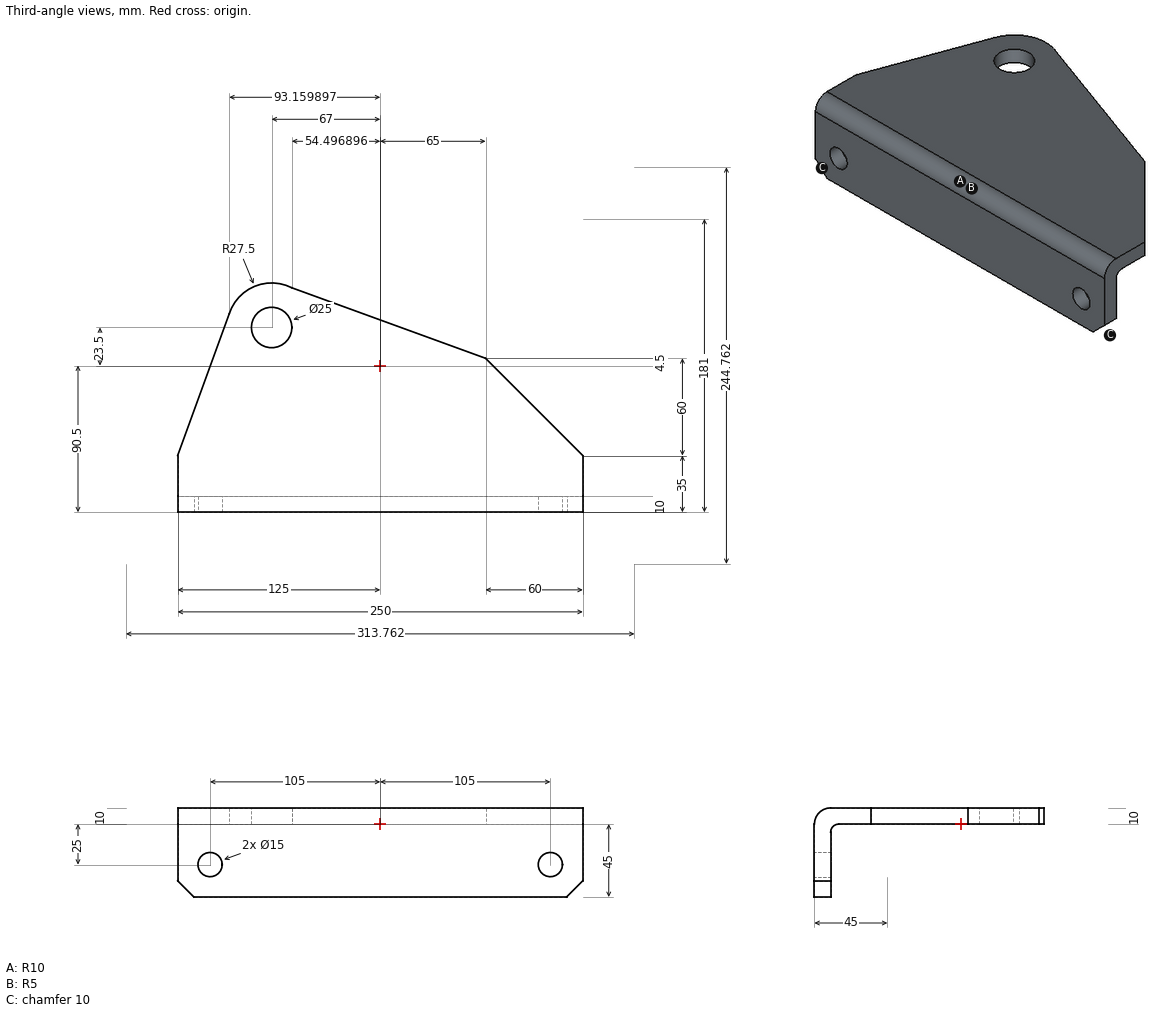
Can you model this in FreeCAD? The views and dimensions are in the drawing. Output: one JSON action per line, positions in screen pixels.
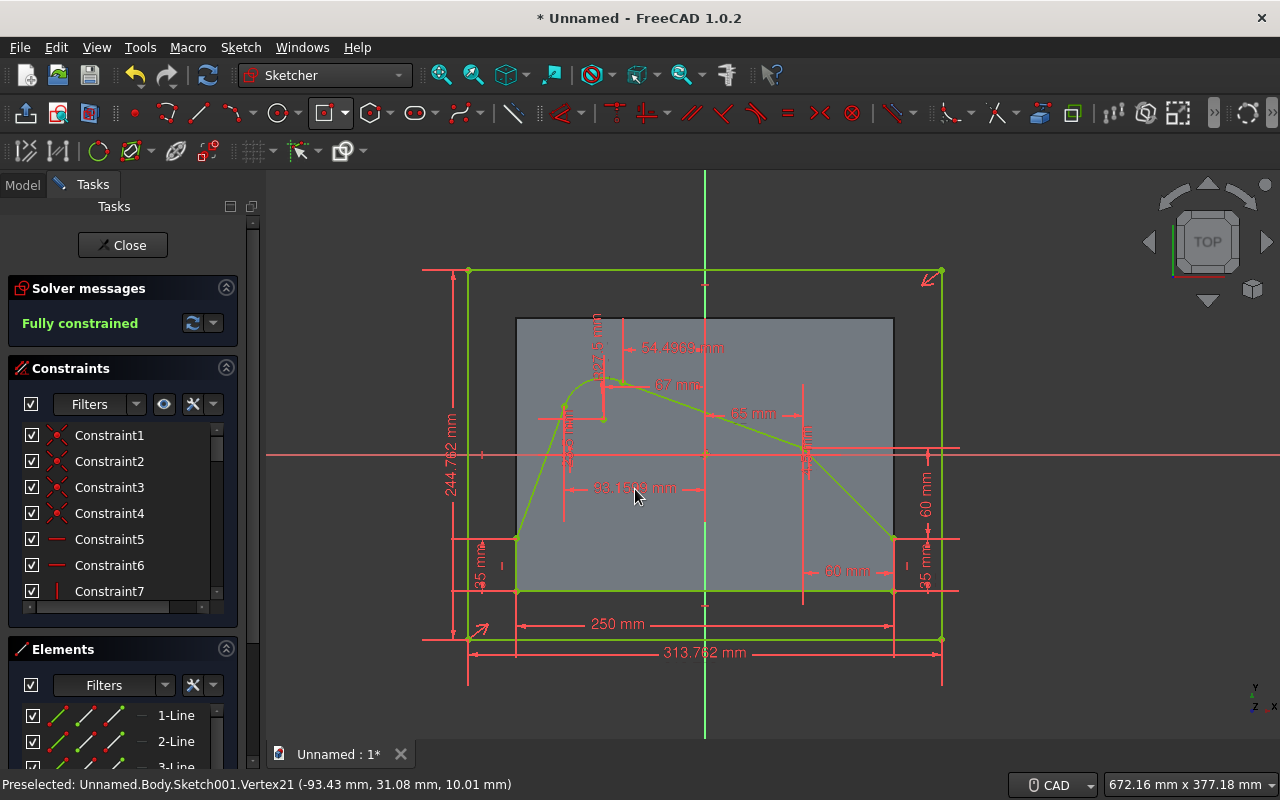
{"action": "left_click", "coordinate": [123, 245]}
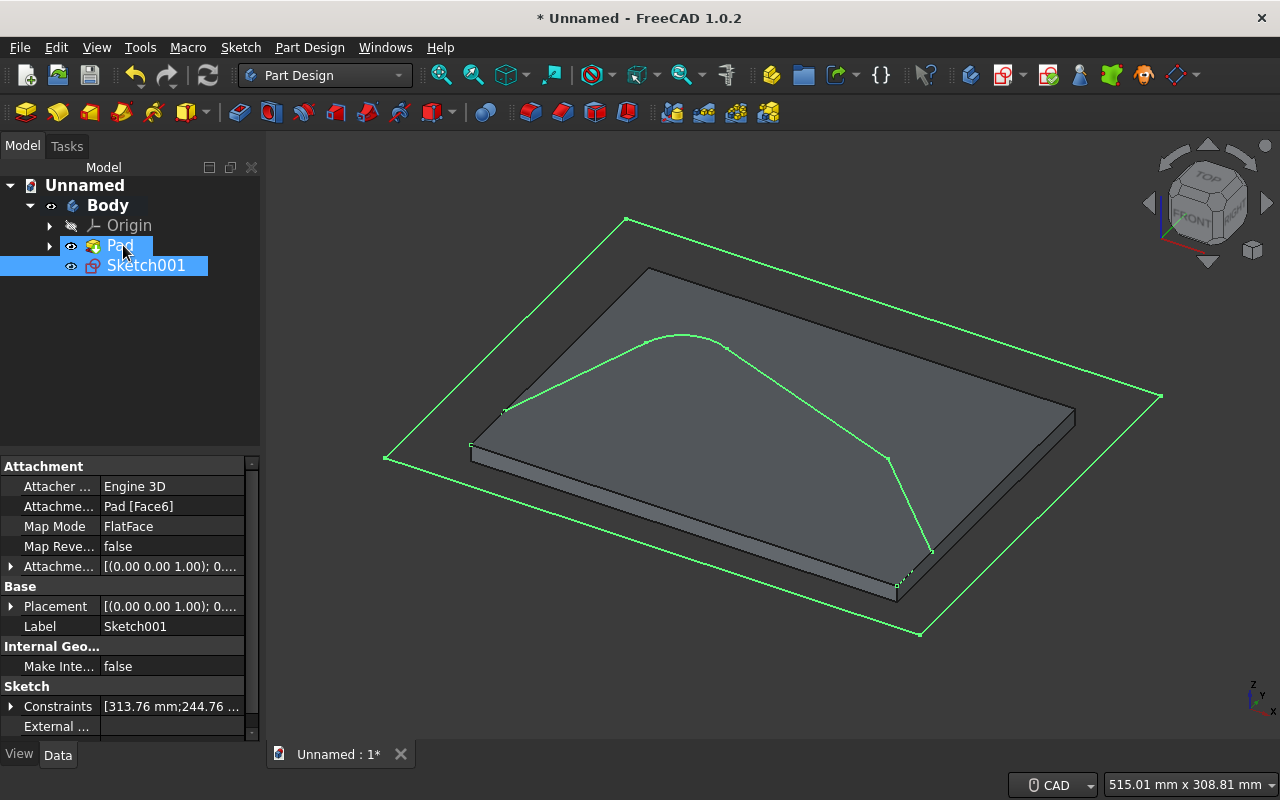
{"action": "left_click", "coordinate": [240, 112]}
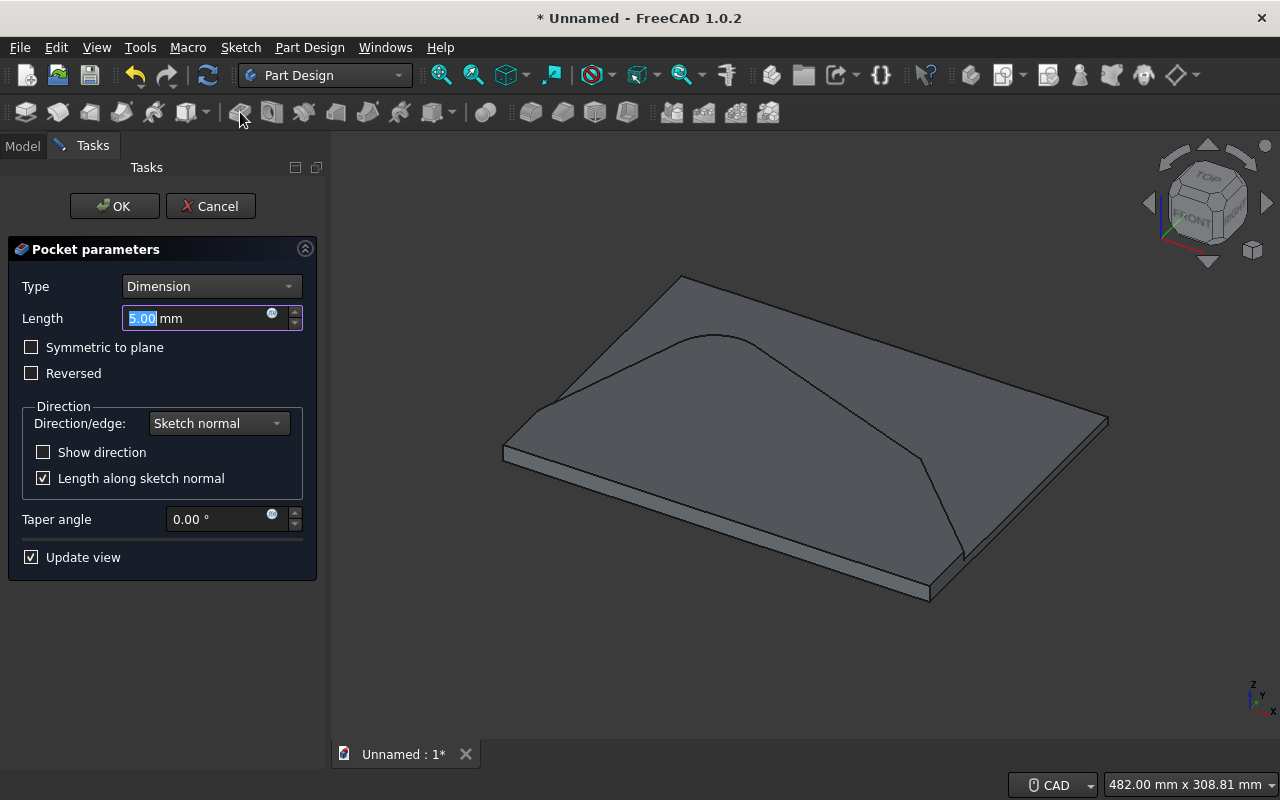
{"action": "type", "text": "10"}
{"action": "key", "text": "Tab"}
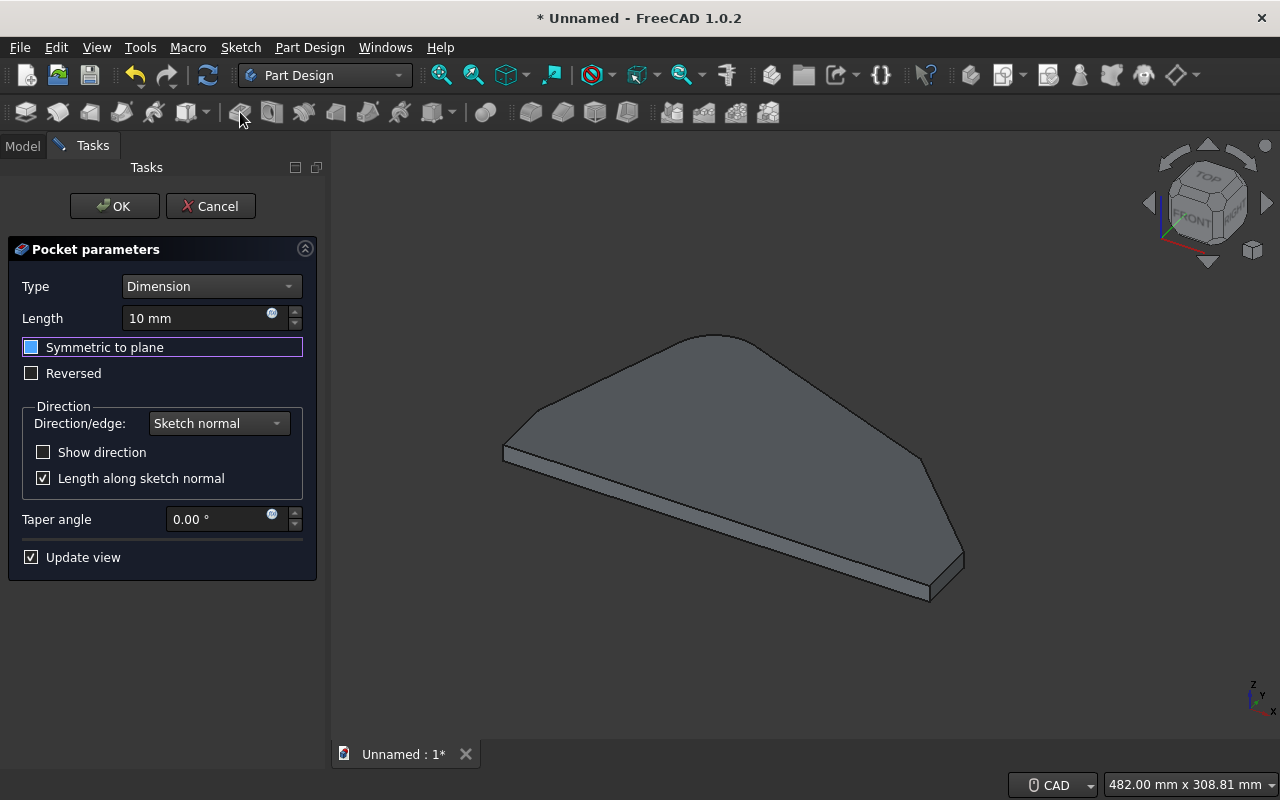
{"action": "left_click", "coordinate": [115, 206]}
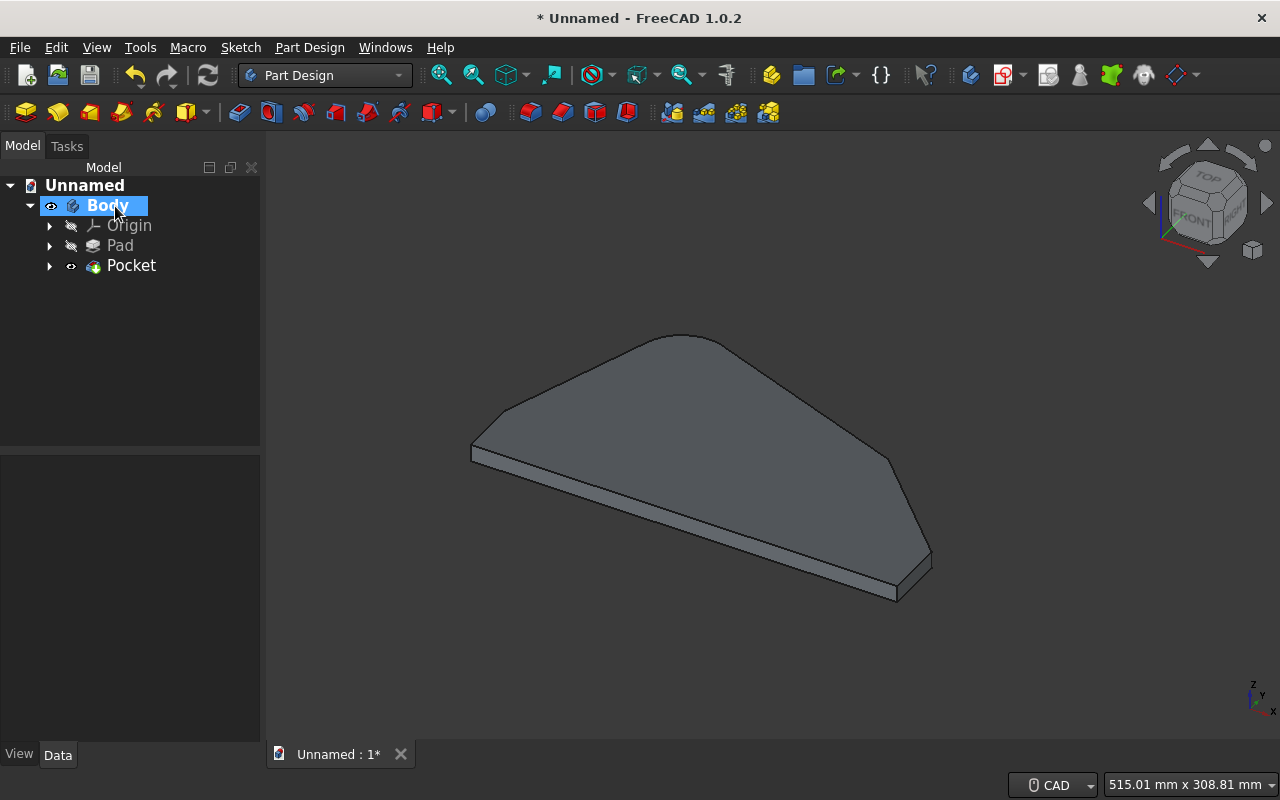
{"action": "left_click", "coordinate": [693, 425]}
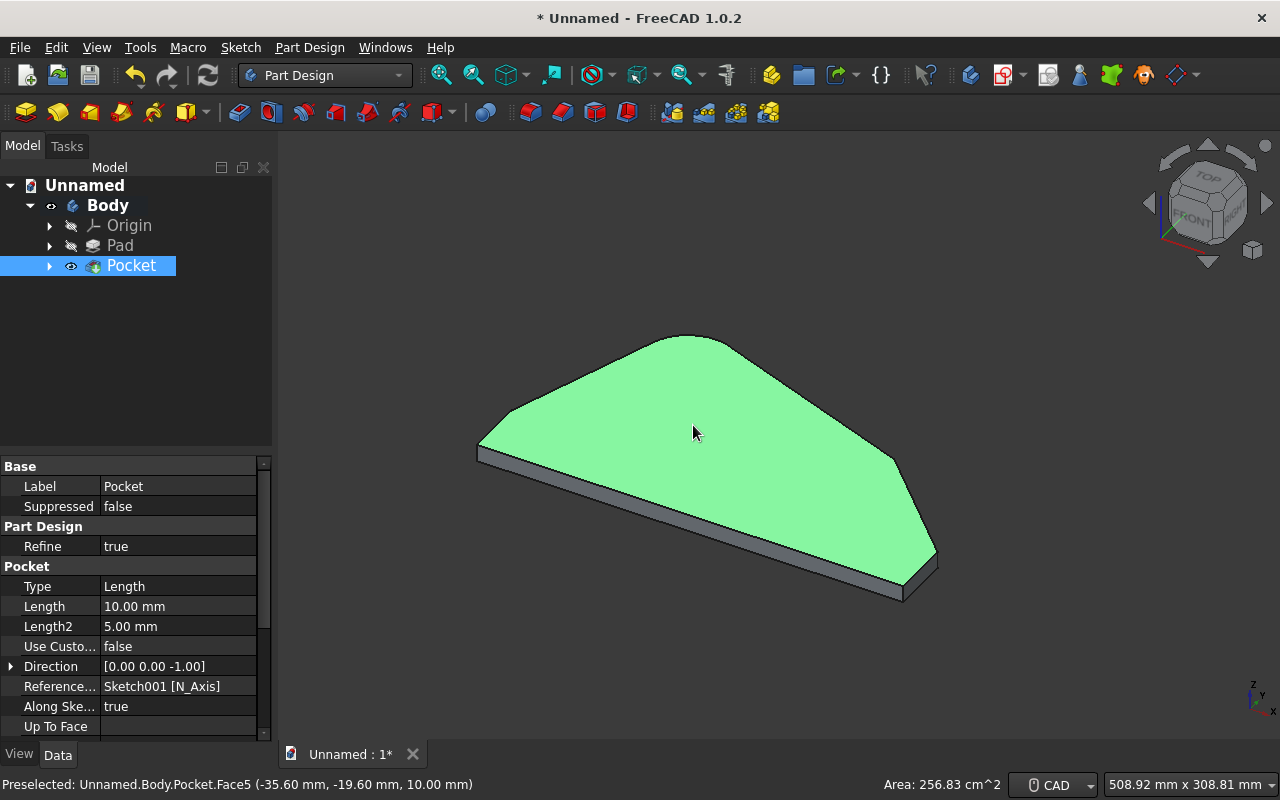
{"action": "left_click", "coordinate": [1004, 76]}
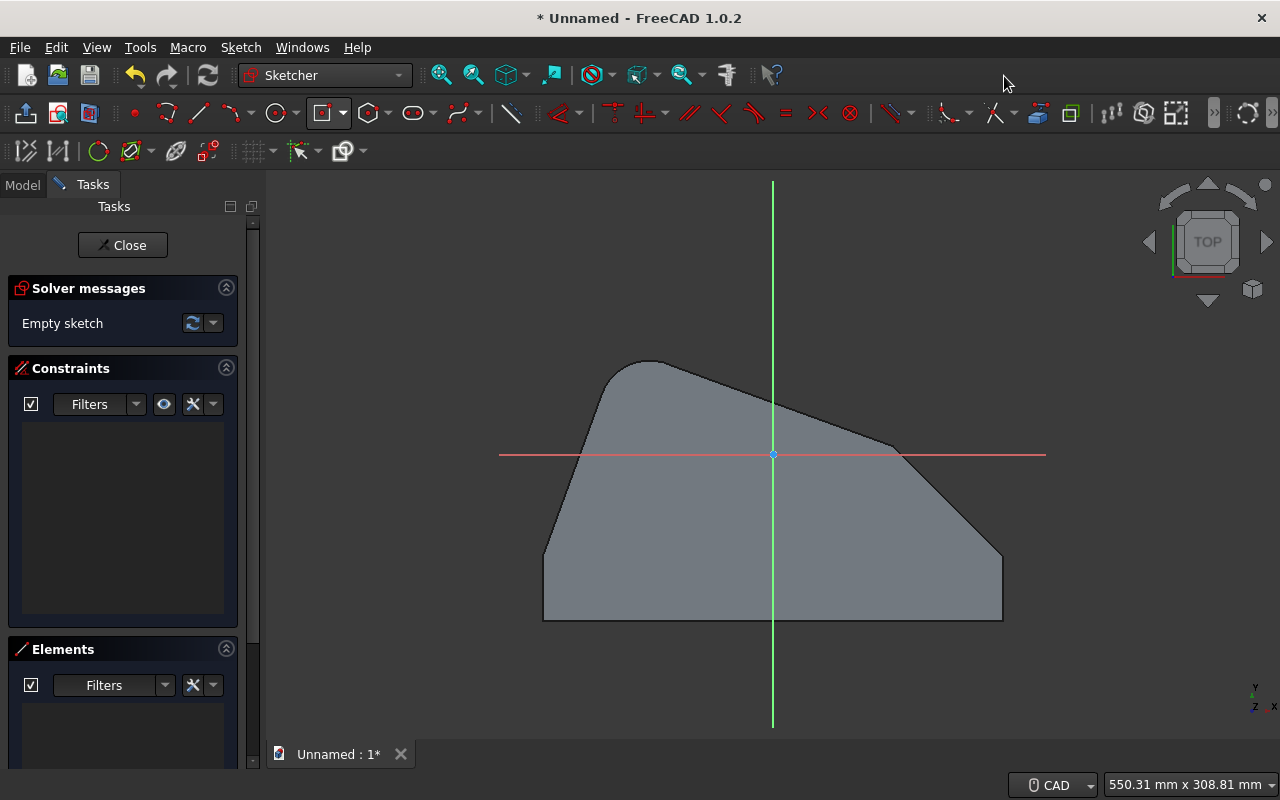
{"action": "scroll", "coordinate": [641, 404], "scroll_direction": "up", "scroll_amount": 10}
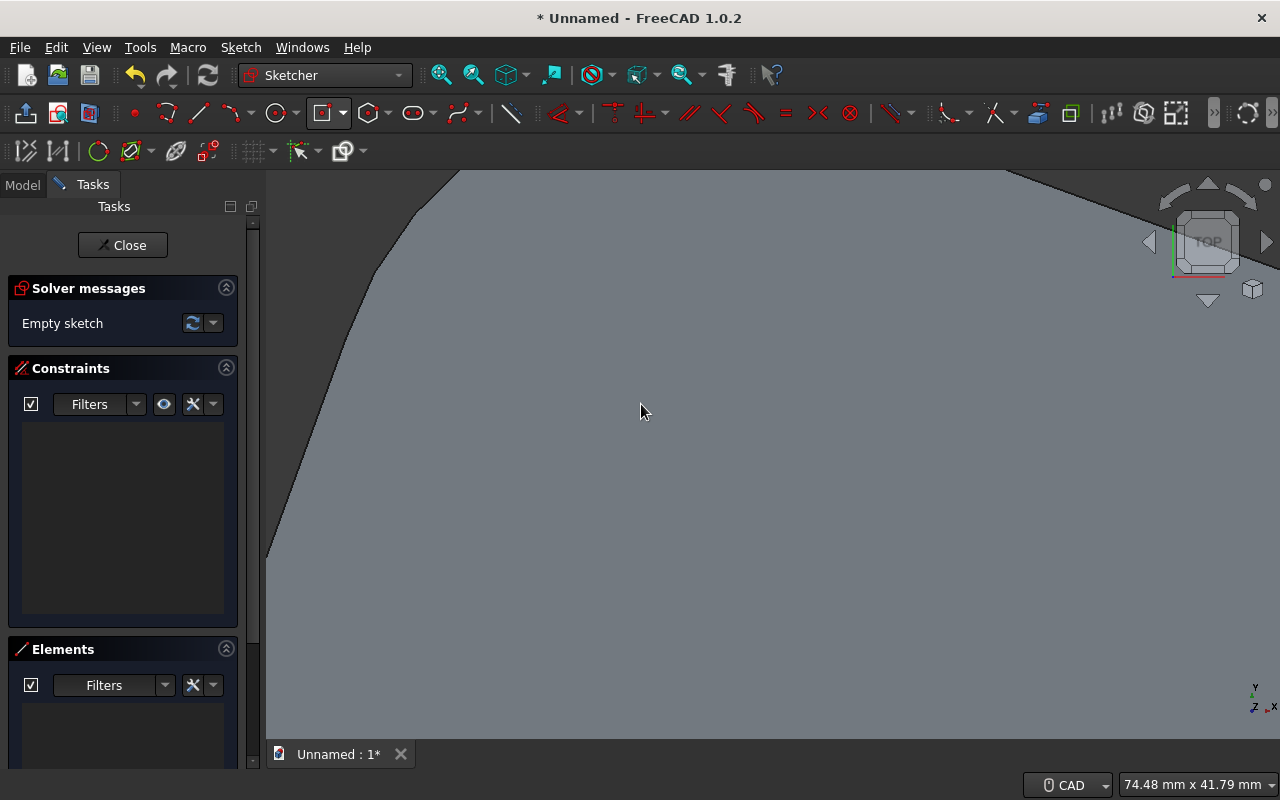
{"action": "key", "text": "g c"}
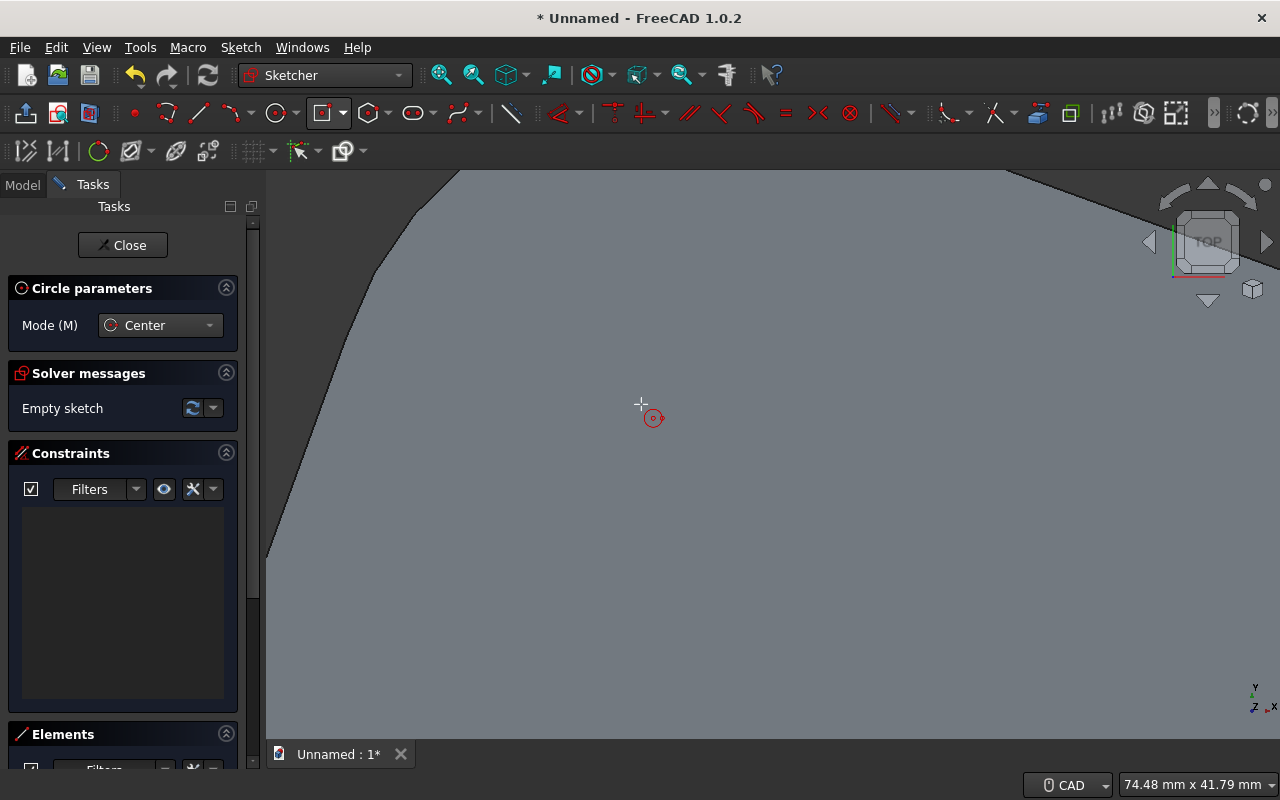
{"action": "left_click", "coordinate": [702, 455]}
{"action": "mouse_move", "coordinate": [822, 334]}